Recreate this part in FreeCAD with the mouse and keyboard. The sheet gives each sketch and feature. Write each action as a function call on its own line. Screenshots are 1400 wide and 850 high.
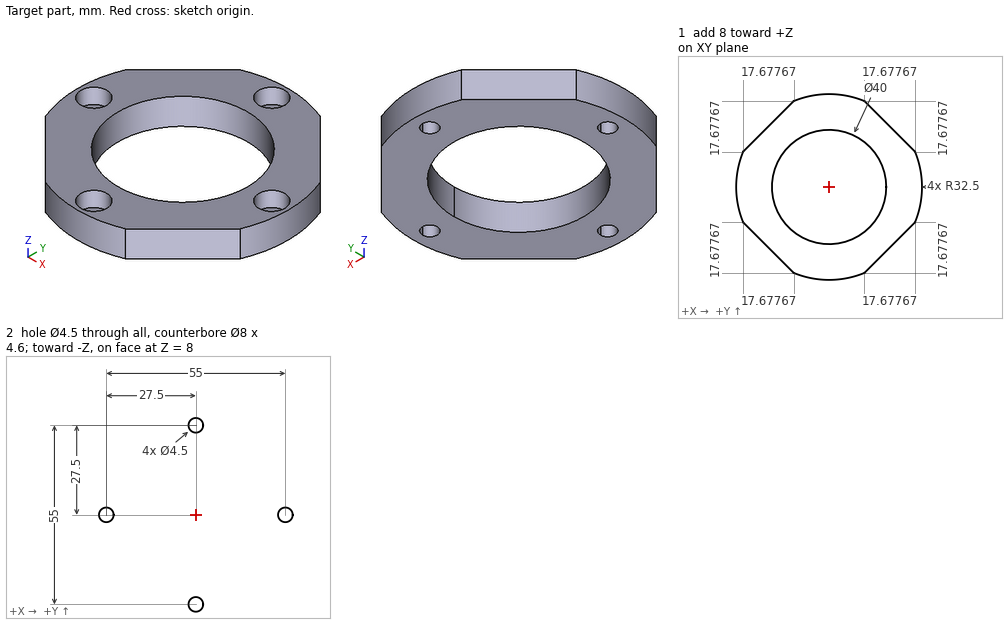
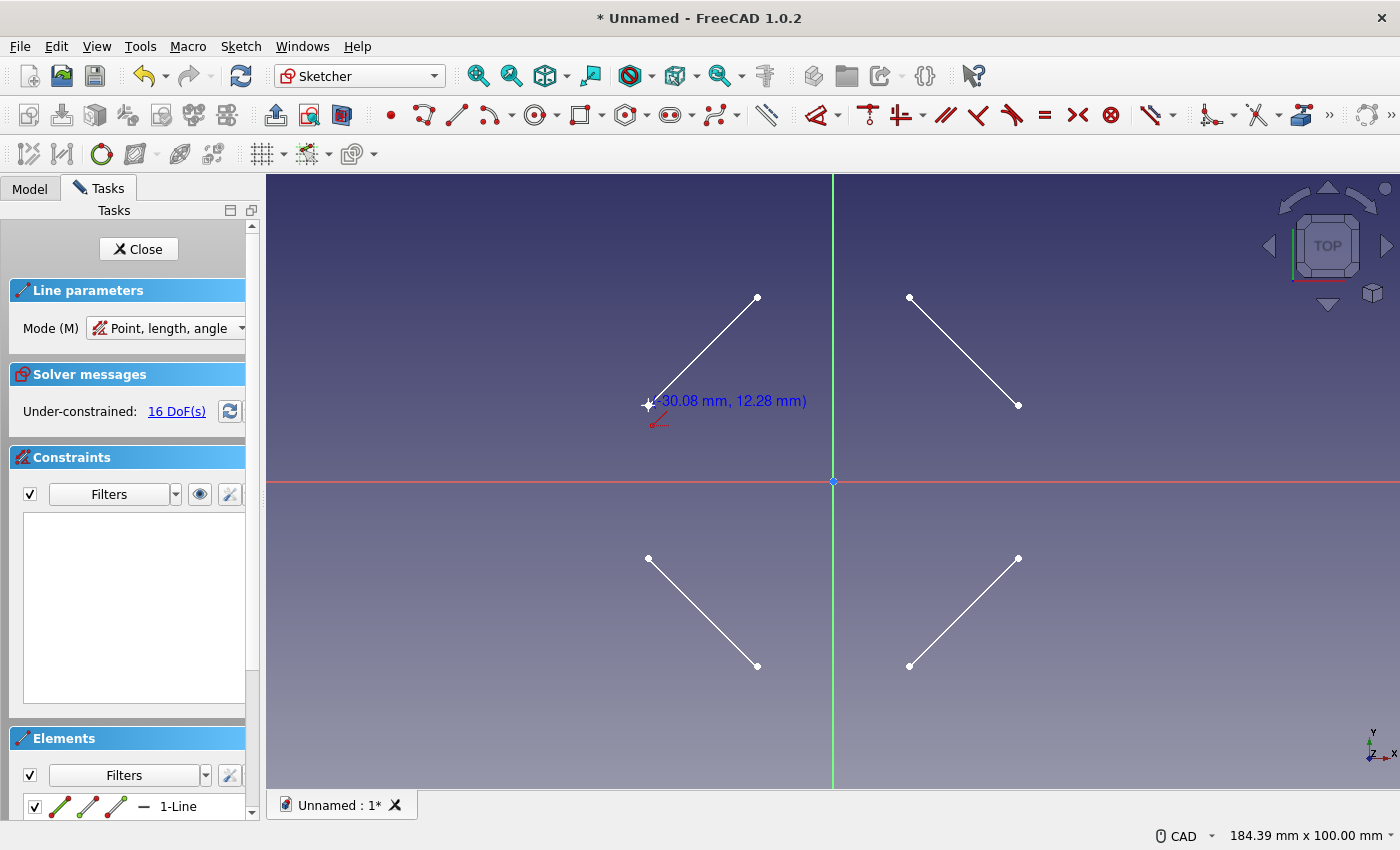
click(512, 116)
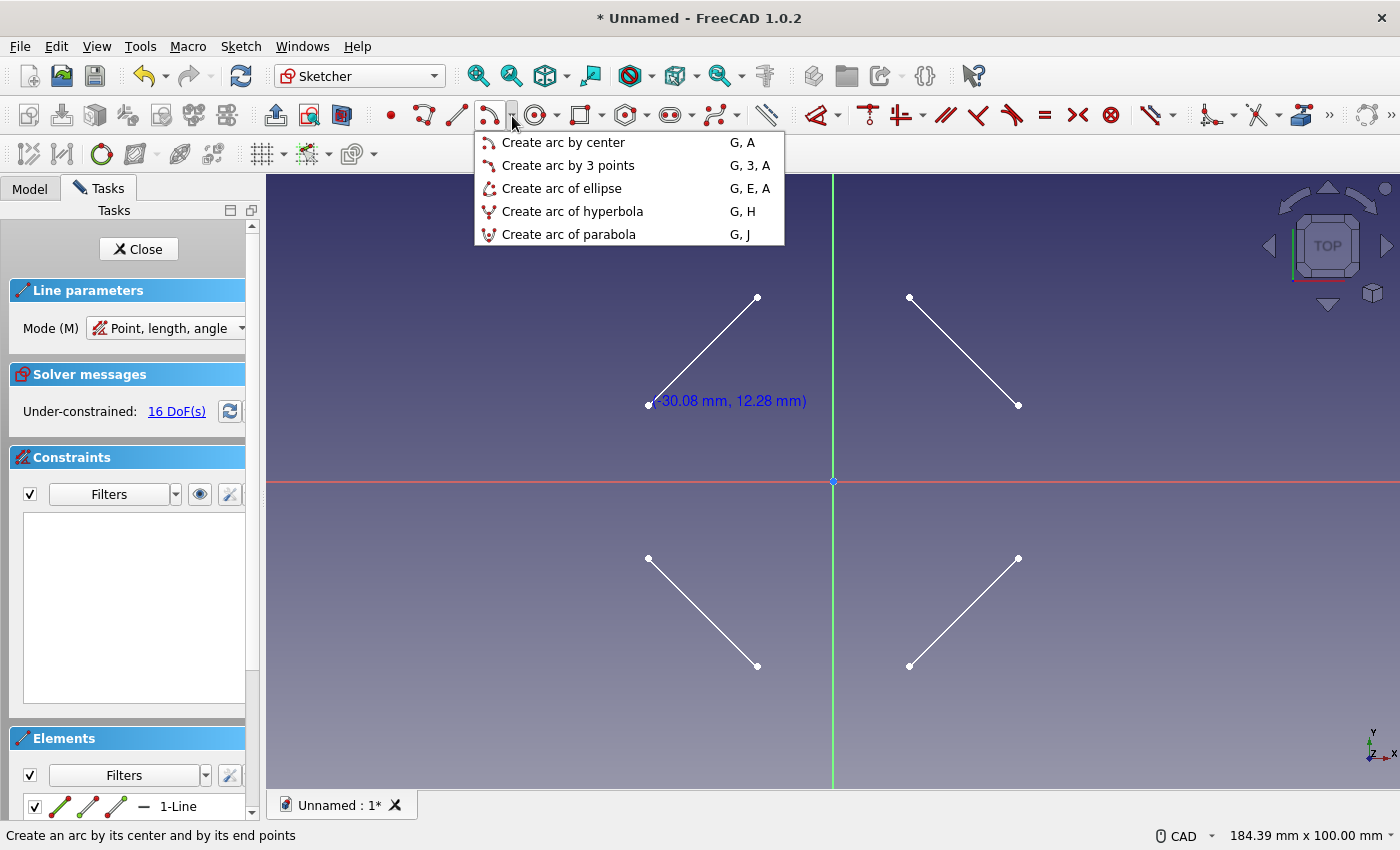
click(630, 166)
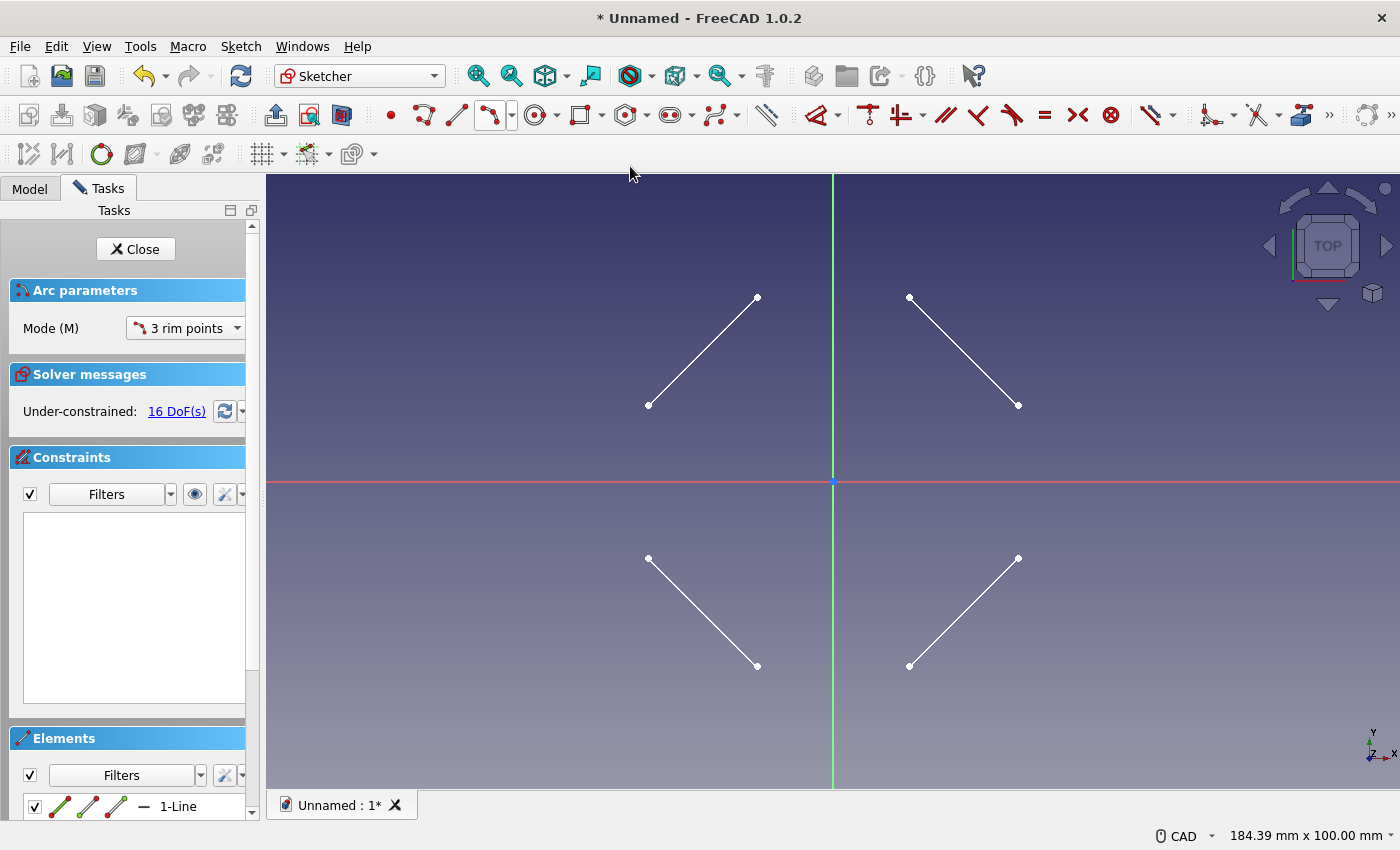
click(757, 667)
click(909, 667)
click(817, 681)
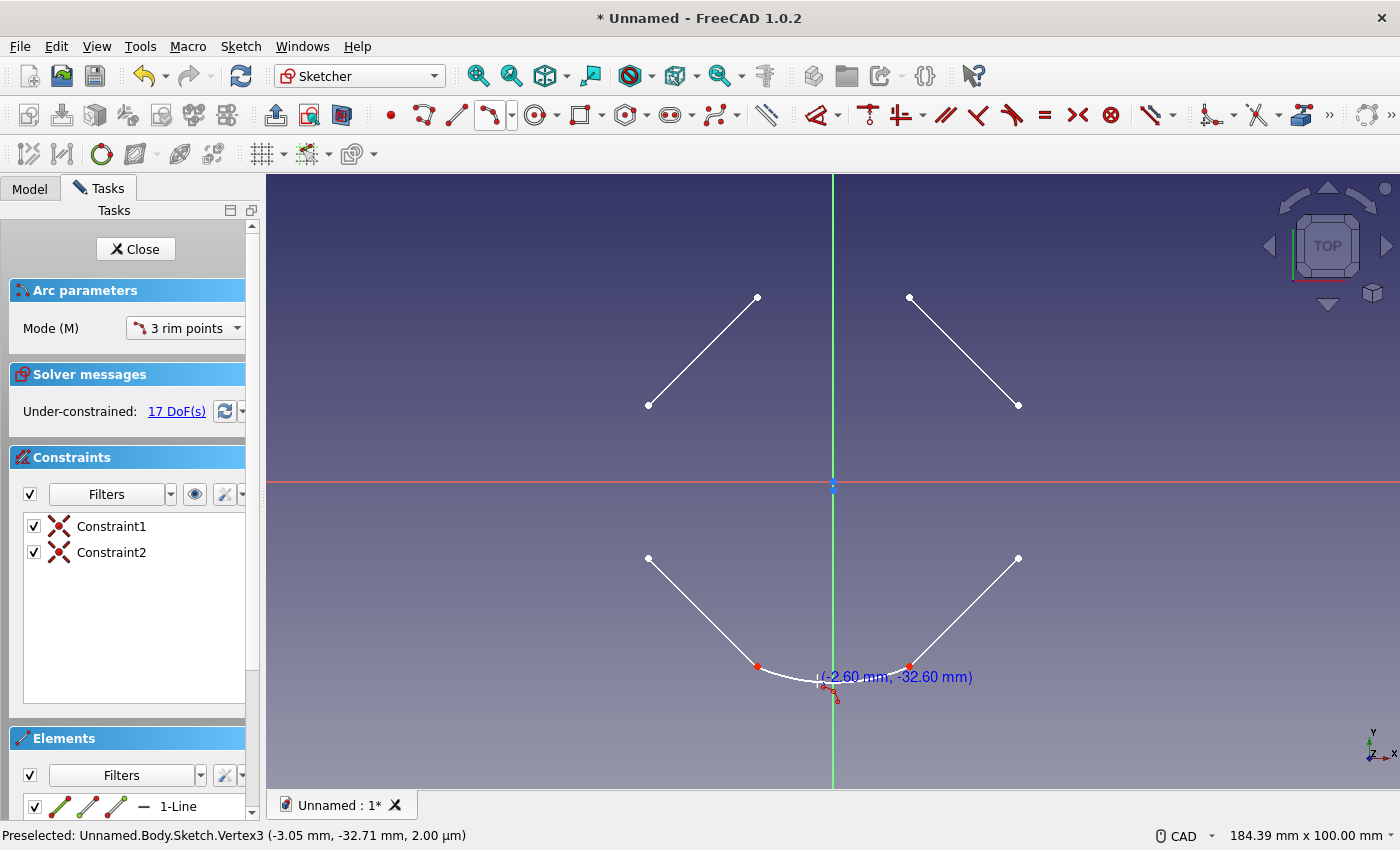
click(1018, 559)
click(1018, 406)
click(1032, 497)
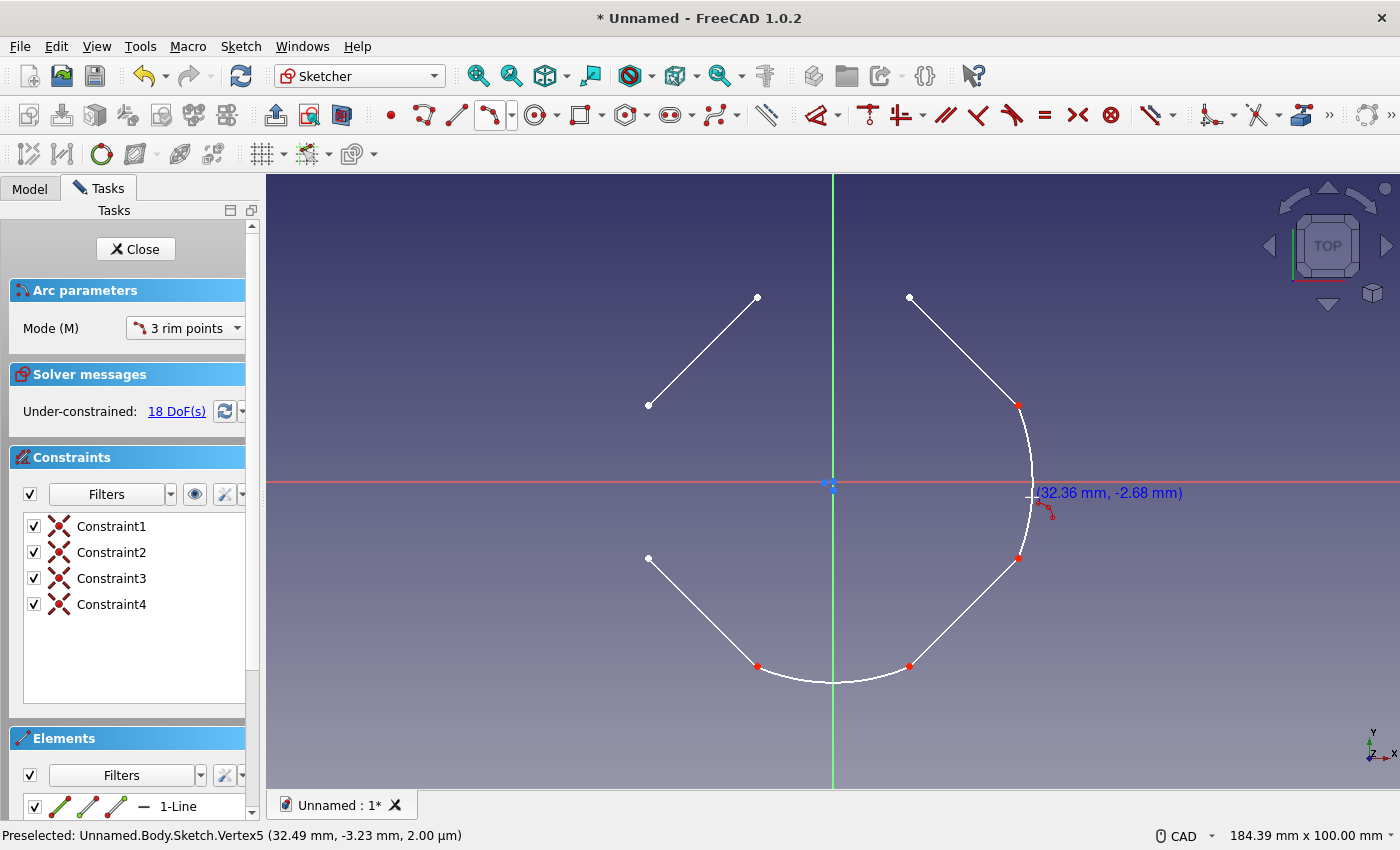
click(909, 298)
click(757, 298)
click(849, 282)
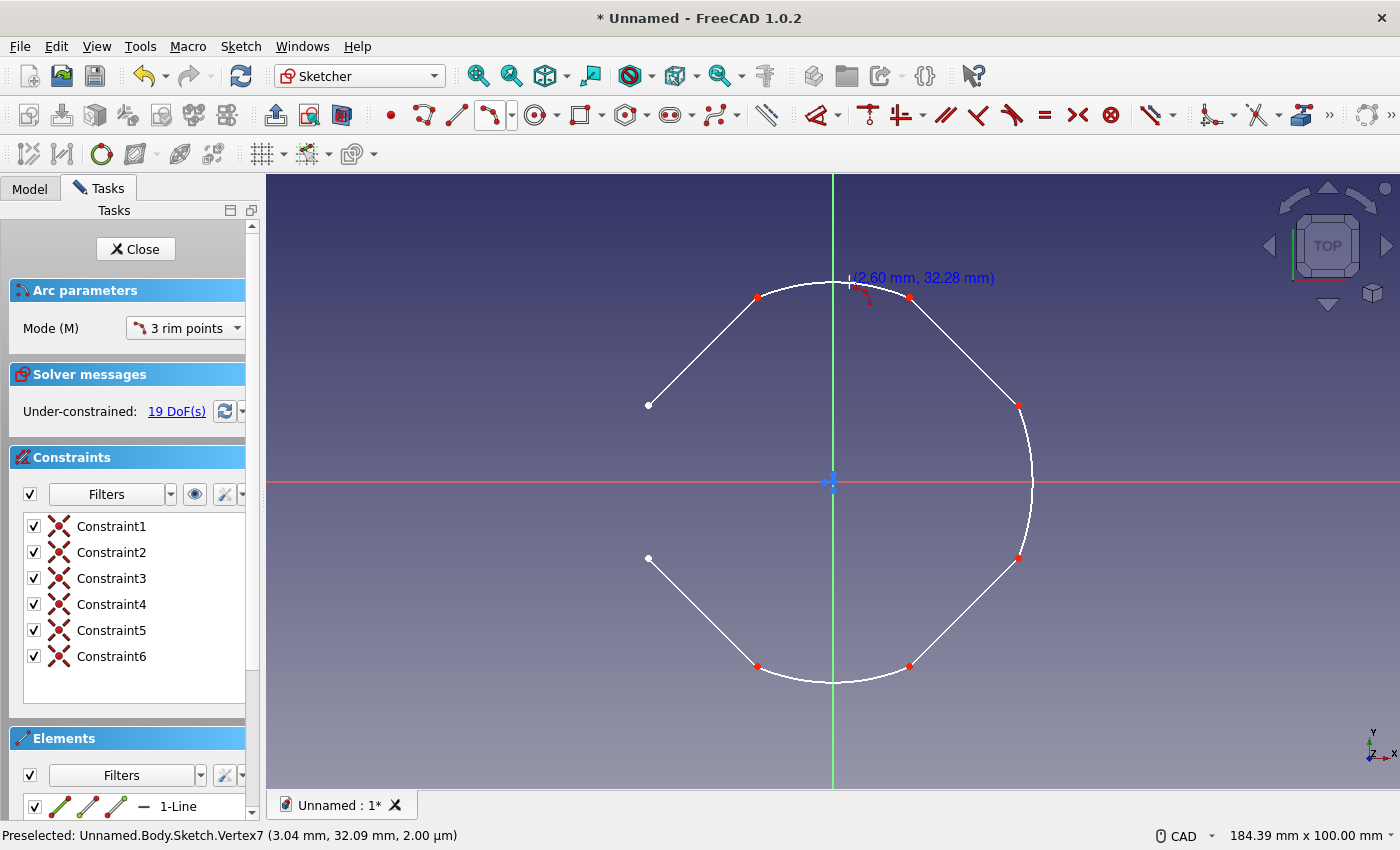
click(648, 406)
click(648, 559)
click(634, 466)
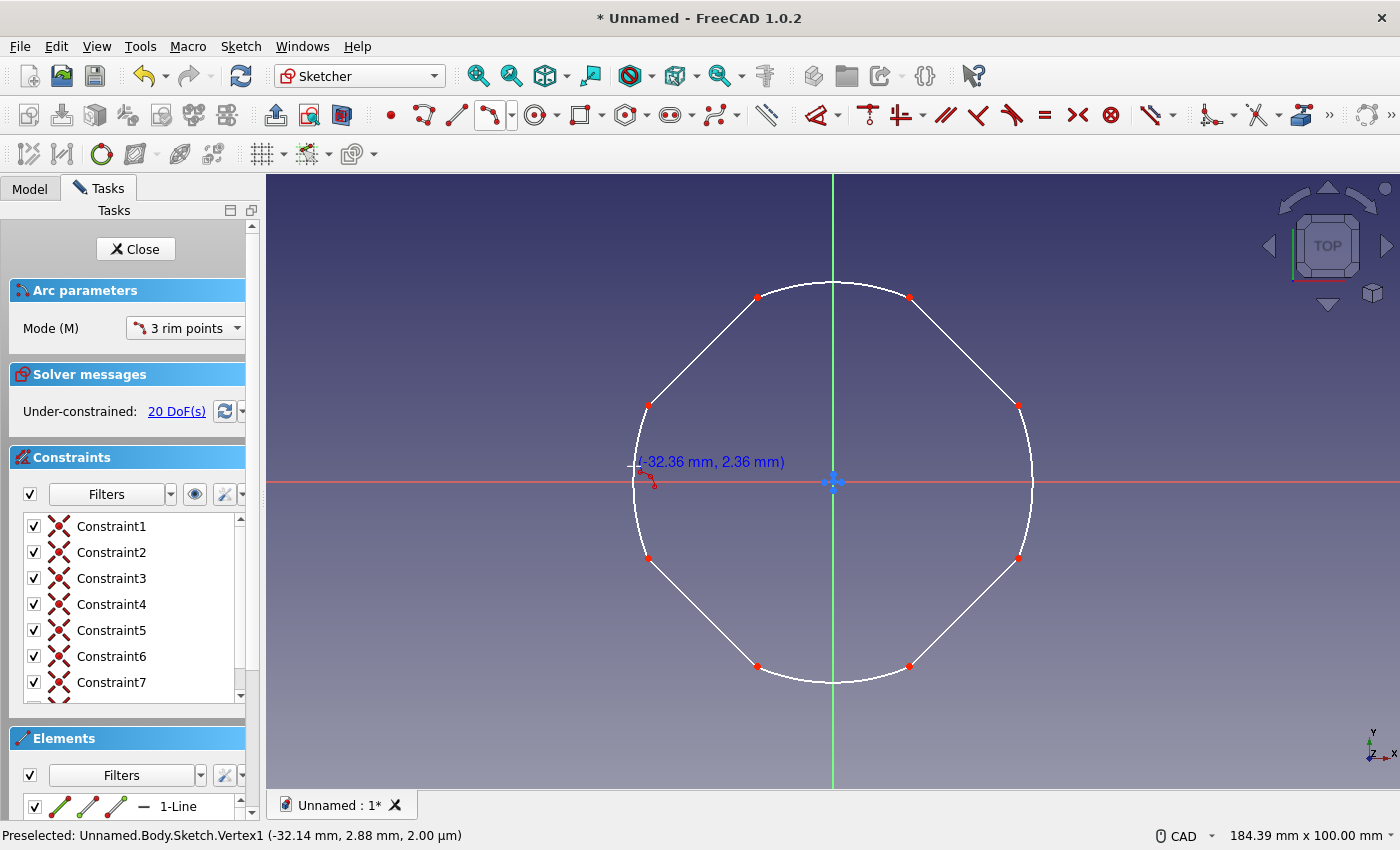
click(534, 116)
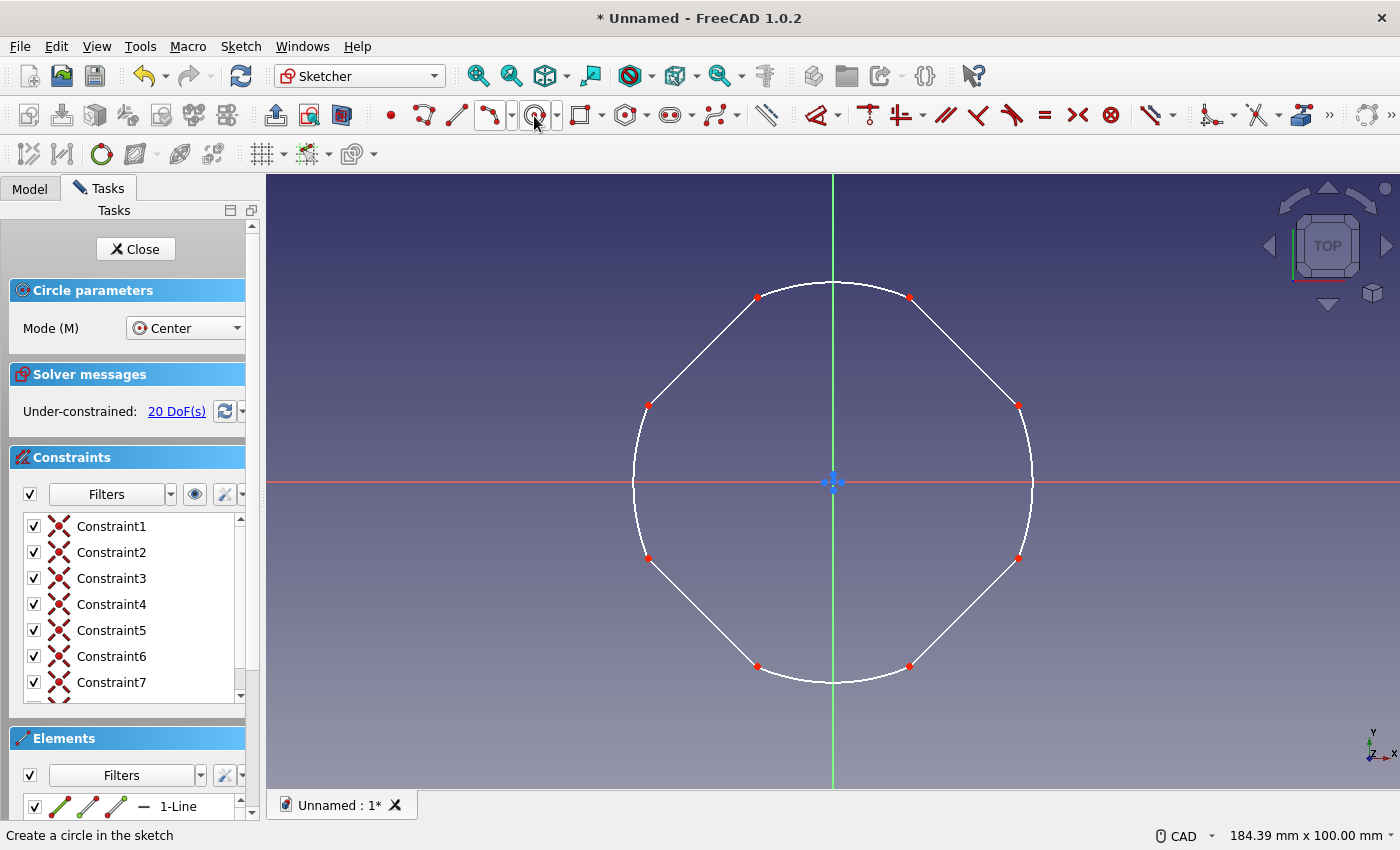
click(833, 482)
move(920, 395)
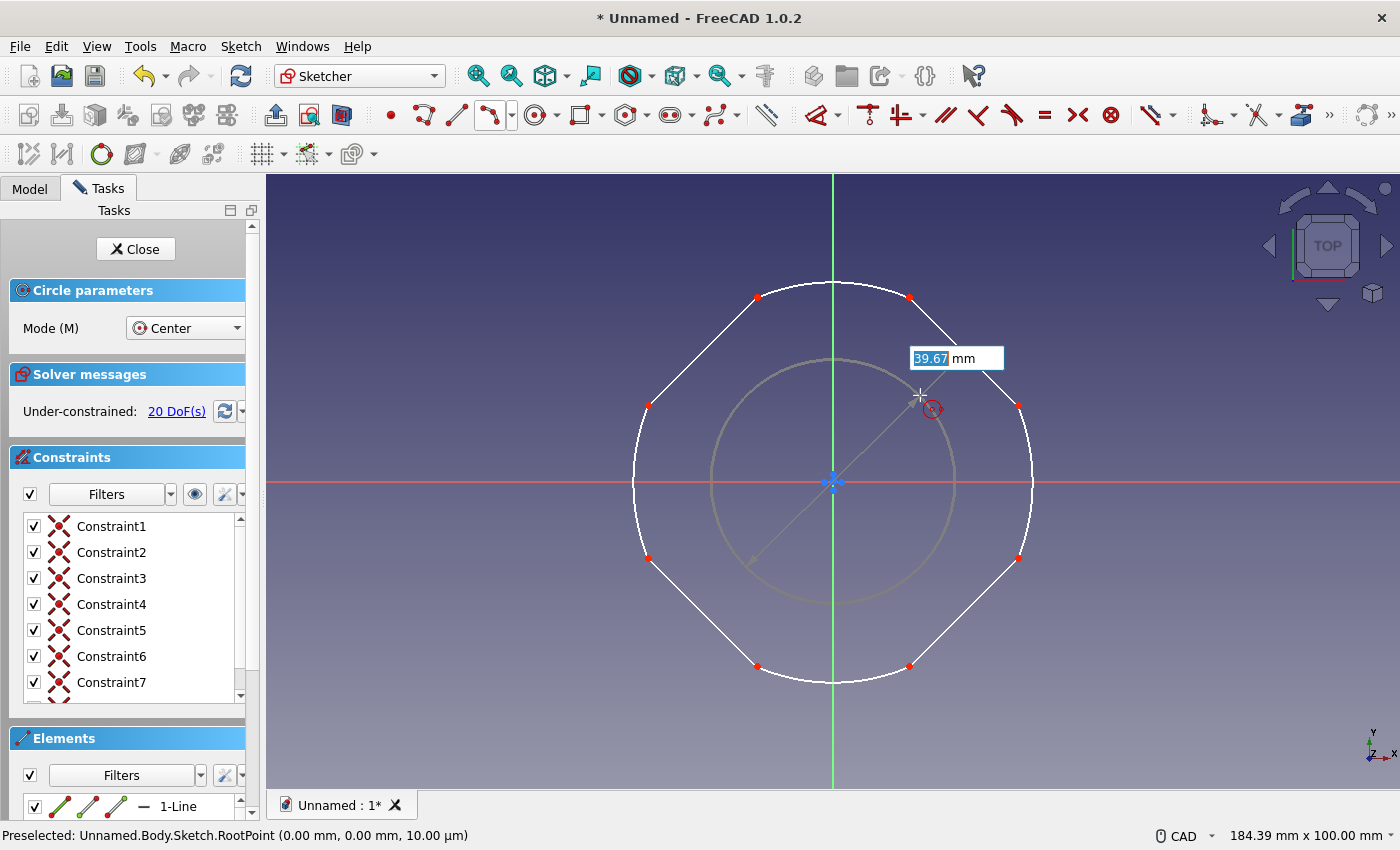
text(40)
key(Return)
key(Escape)